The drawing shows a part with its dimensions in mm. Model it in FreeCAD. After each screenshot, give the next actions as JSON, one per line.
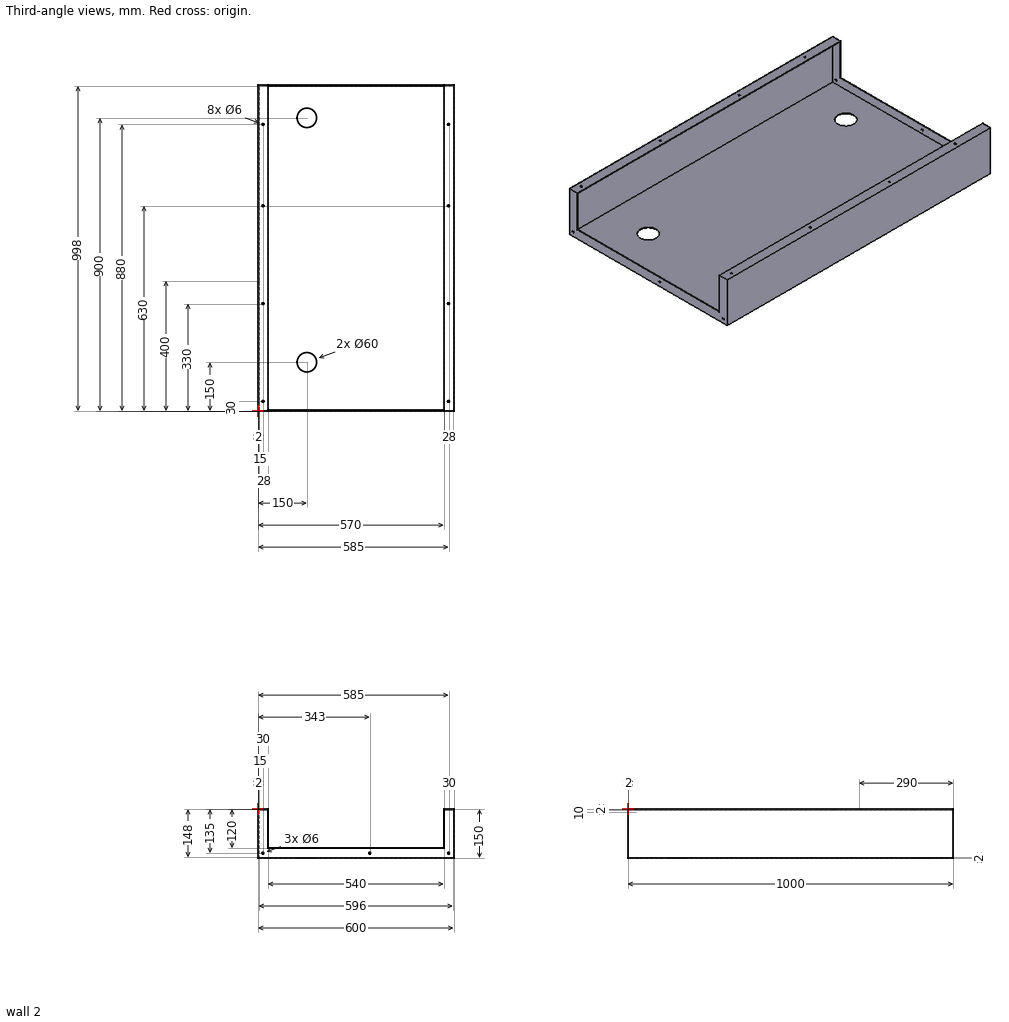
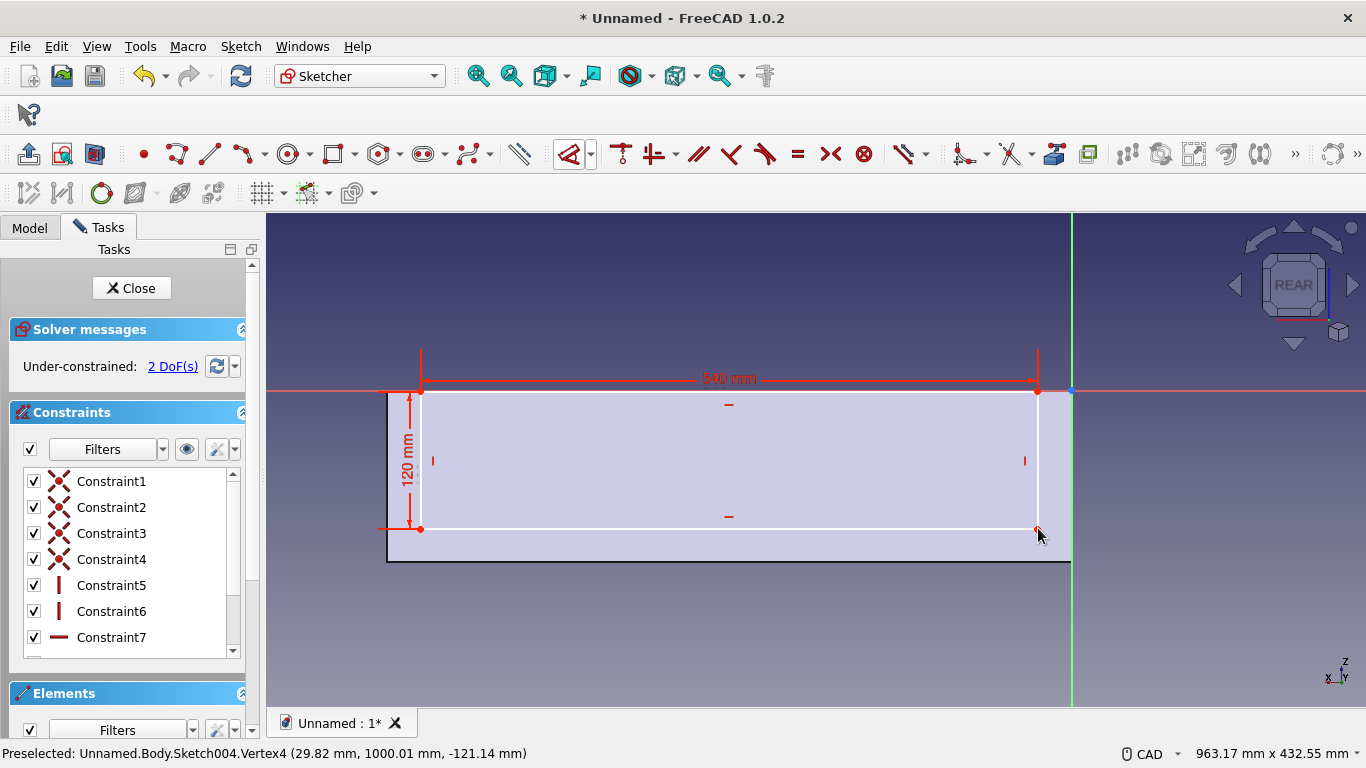
{"action": "left_click", "coordinate": [421, 392]}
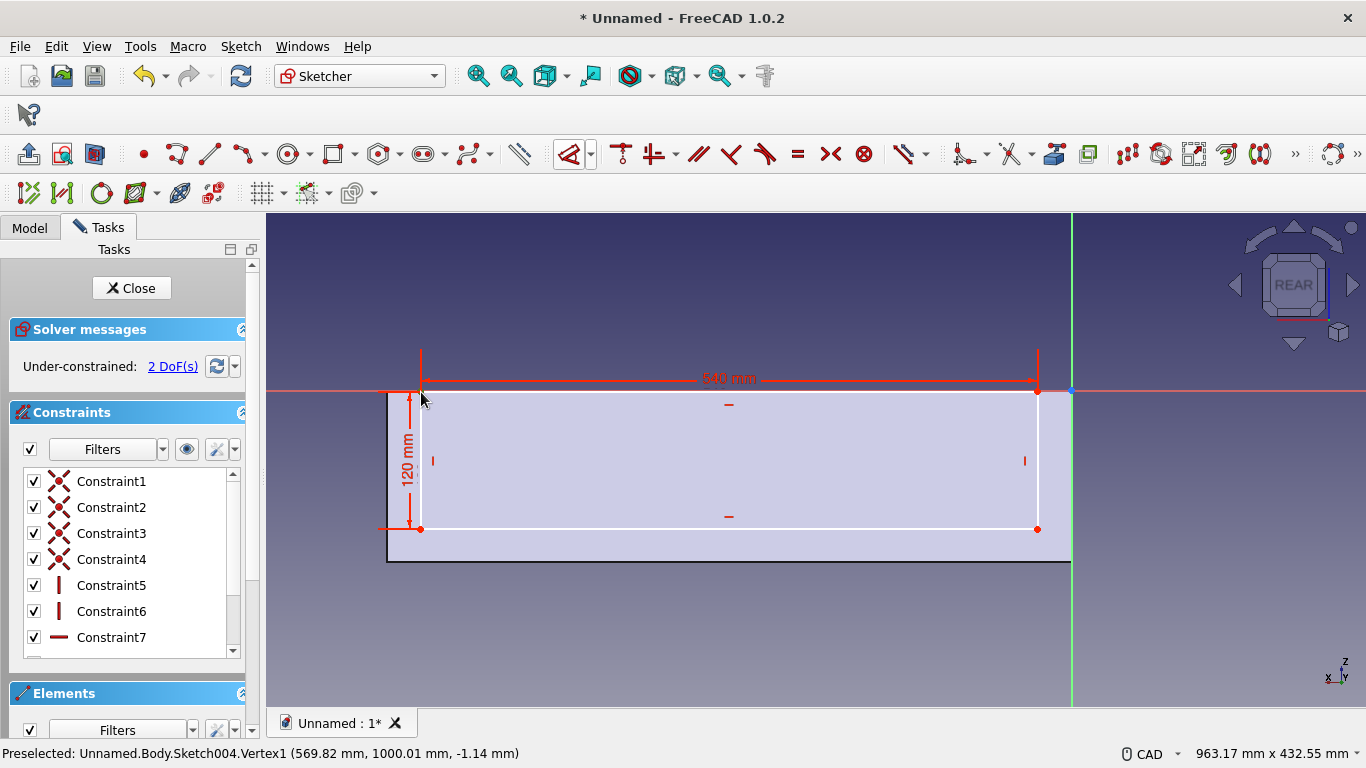
{"action": "left_click", "coordinate": [359, 391]}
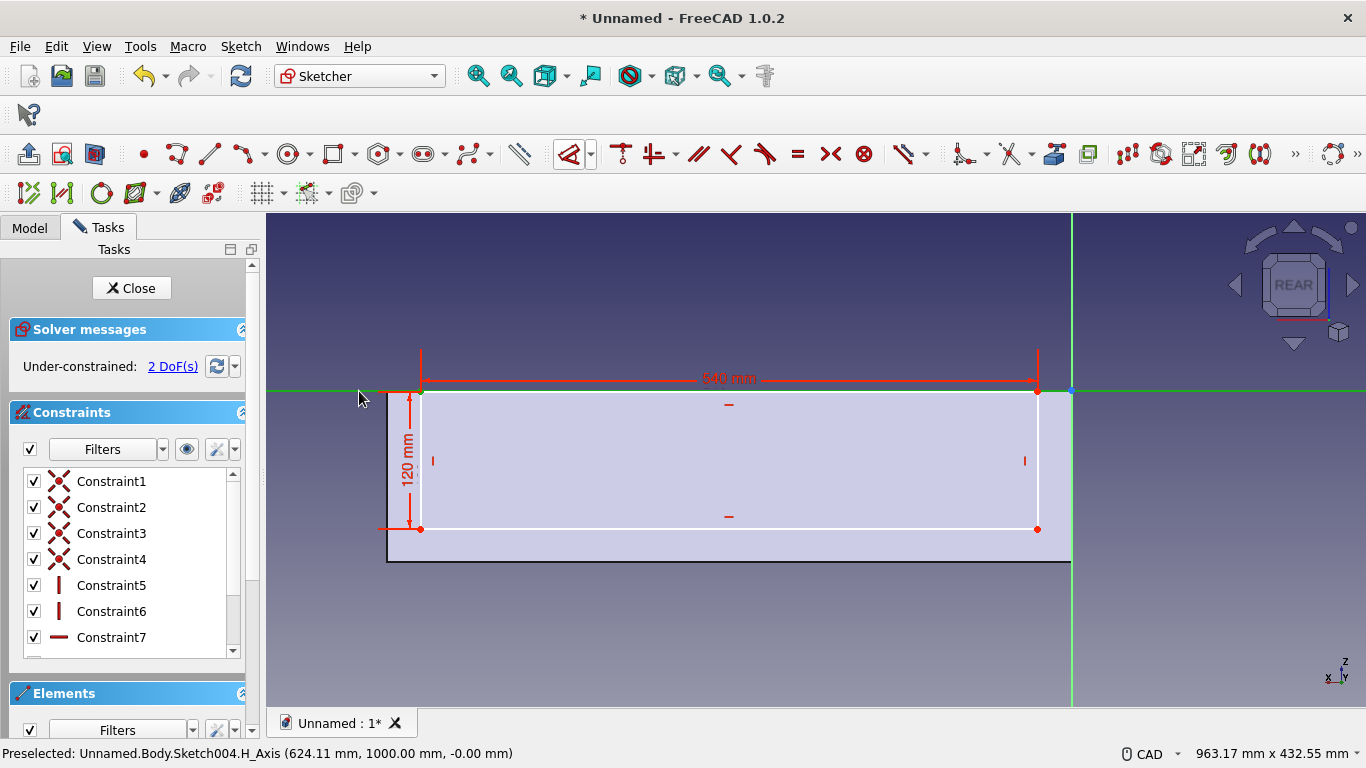
{"action": "left_click", "coordinate": [621, 154]}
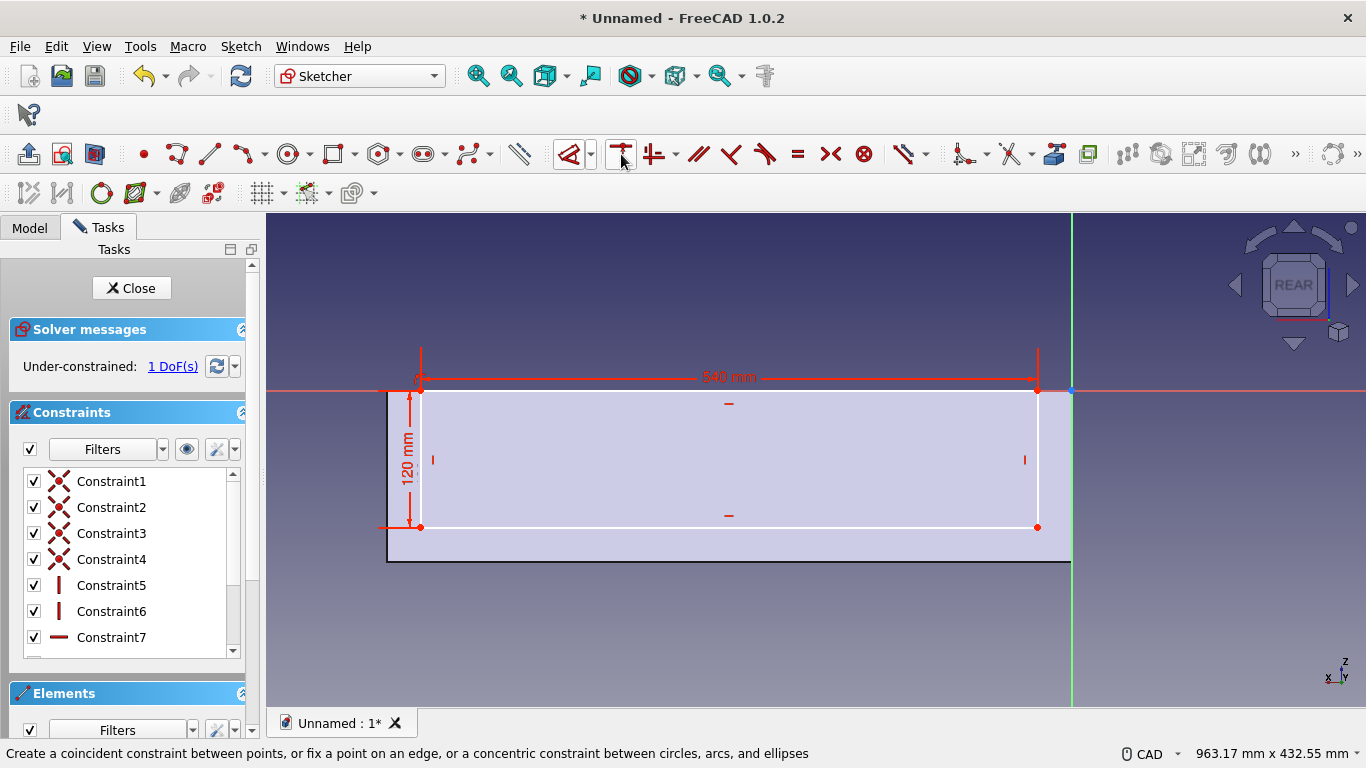
{"action": "left_click", "coordinate": [1038, 528]}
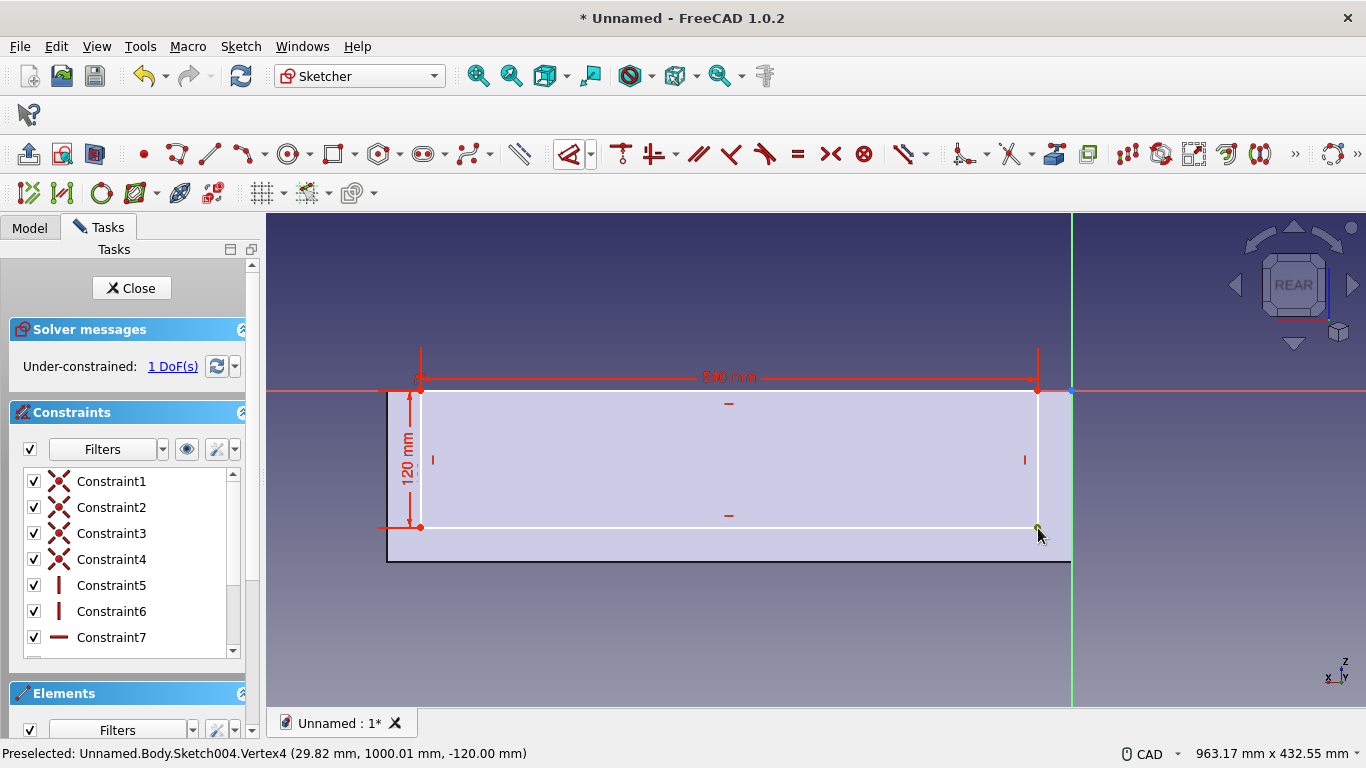
{"action": "left_click", "coordinate": [590, 154]}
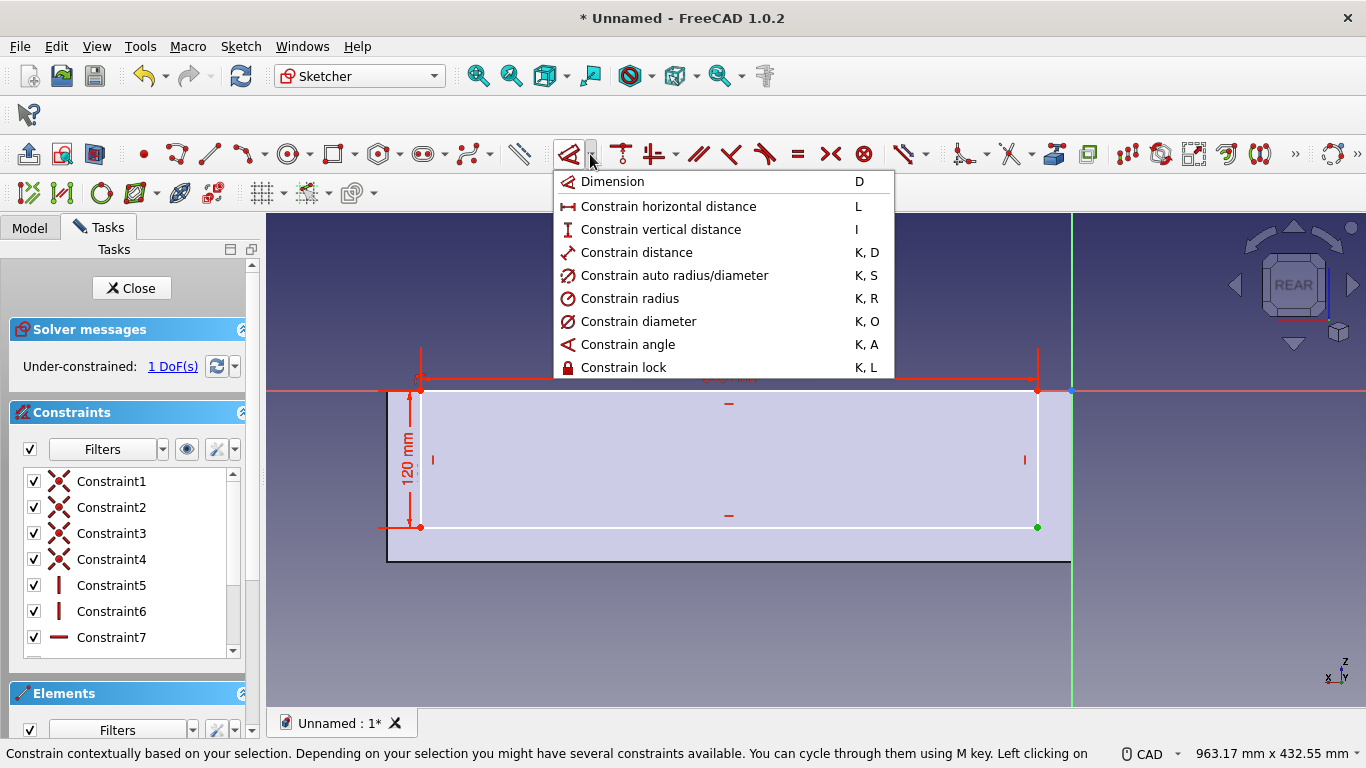
{"action": "left_click", "coordinate": [724, 206]}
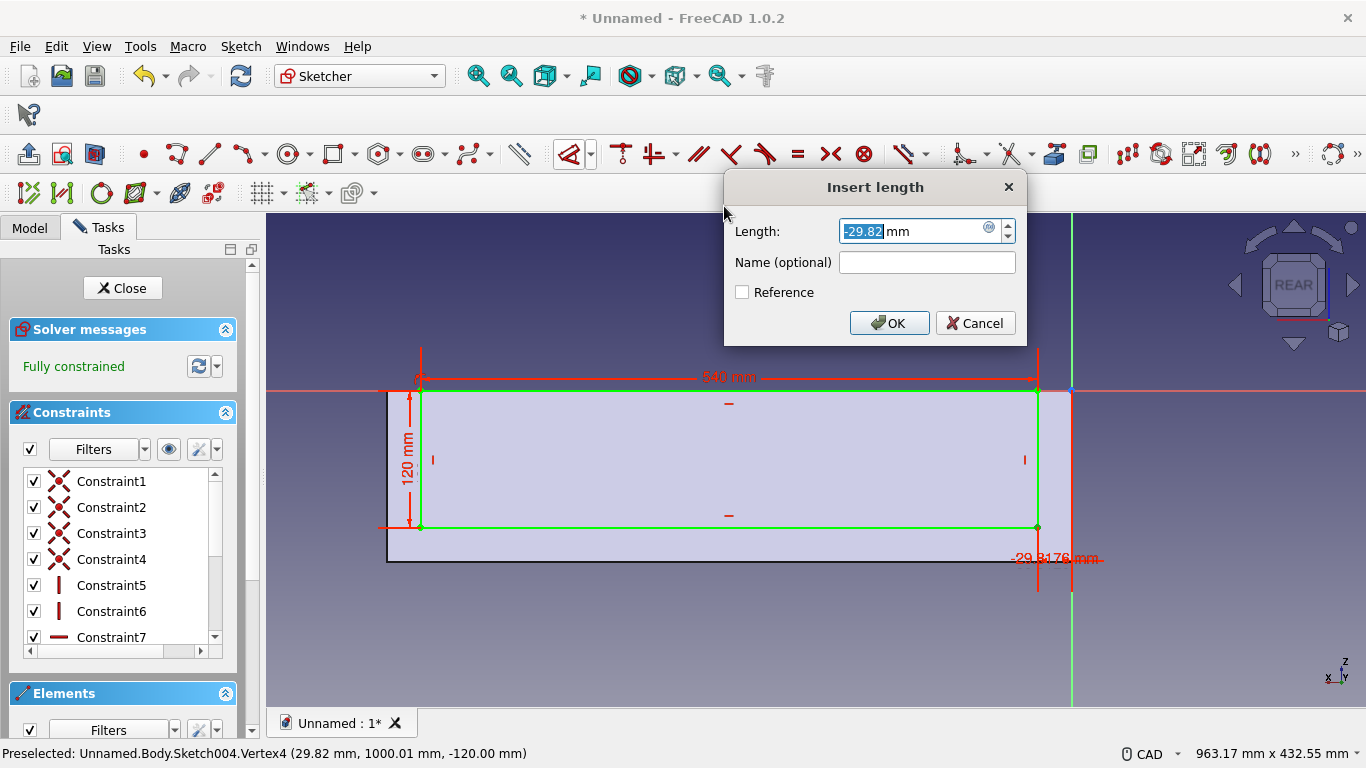
{"action": "type", "text": "-30"}
{"action": "key", "text": "Return"}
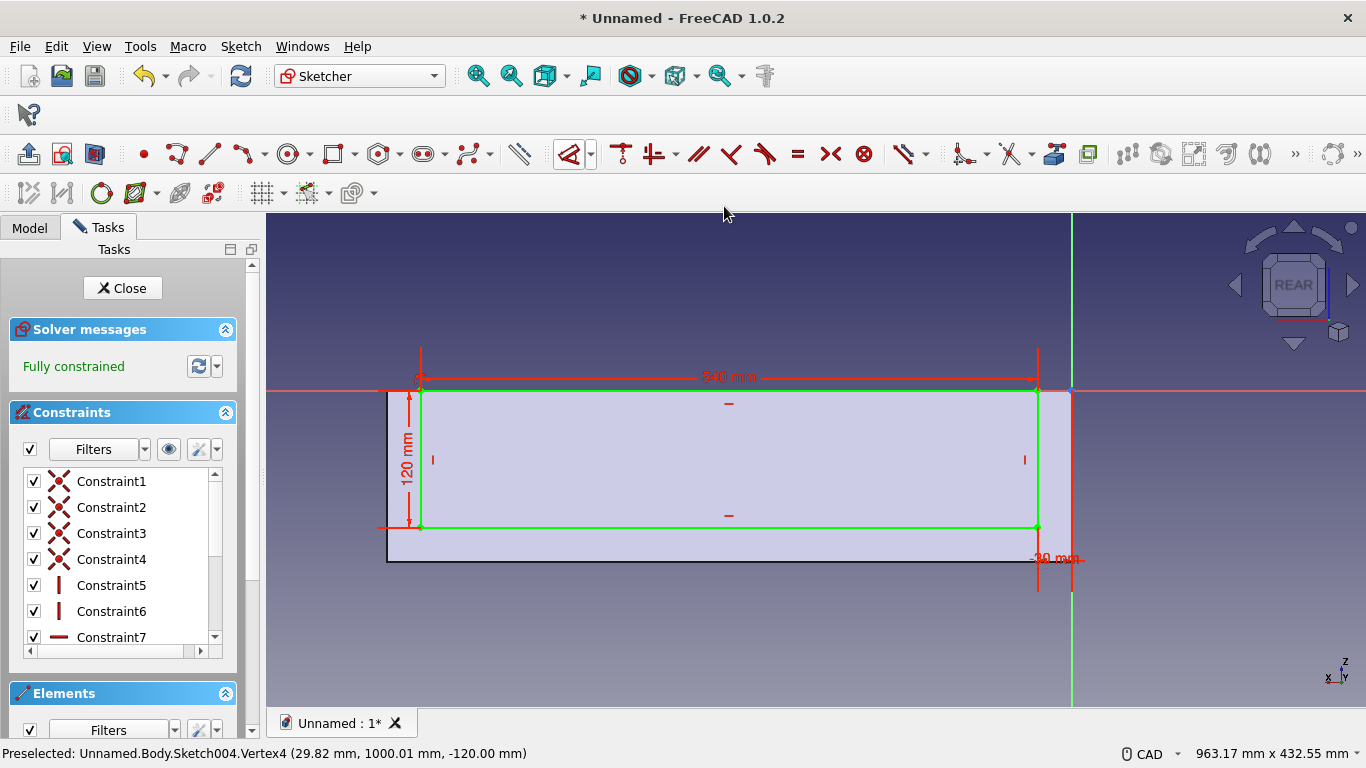
{"action": "left_click", "coordinate": [123, 288]}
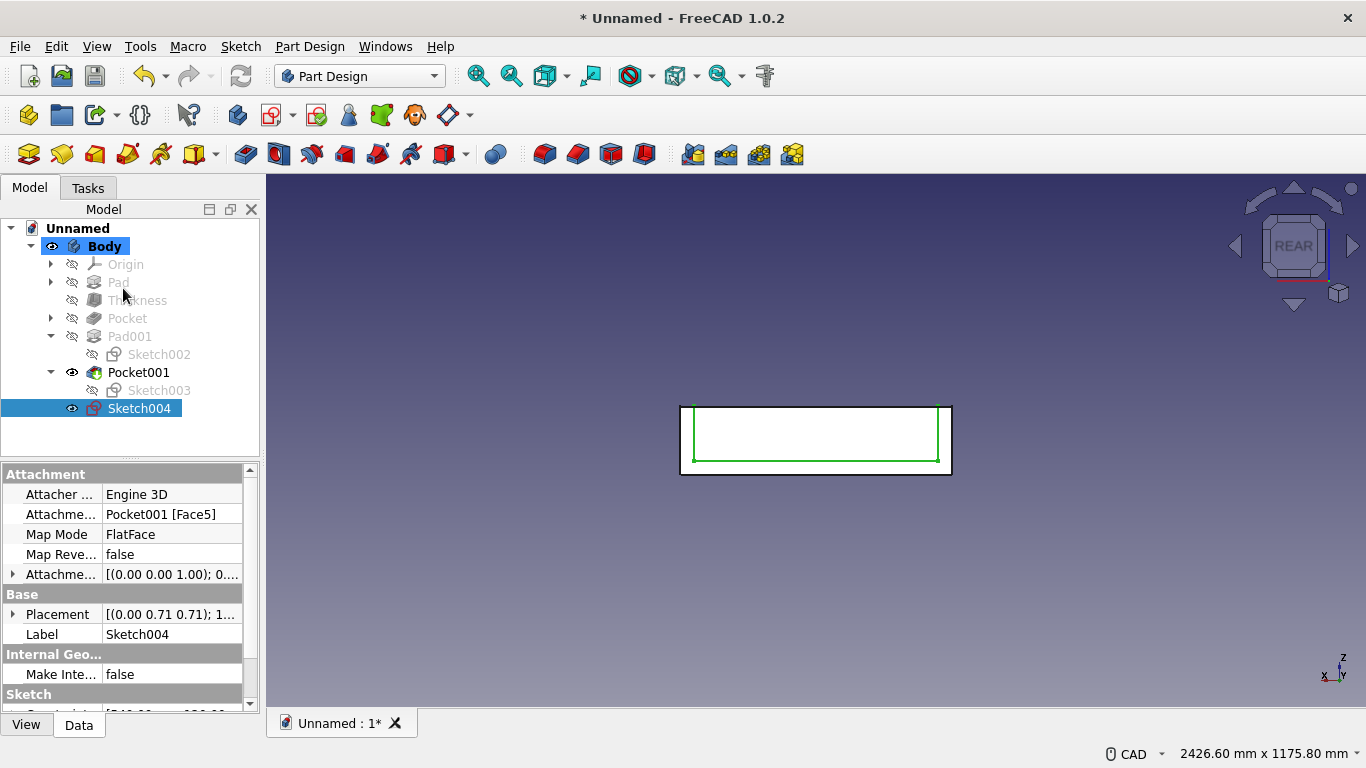
{"action": "left_click", "coordinate": [246, 154]}